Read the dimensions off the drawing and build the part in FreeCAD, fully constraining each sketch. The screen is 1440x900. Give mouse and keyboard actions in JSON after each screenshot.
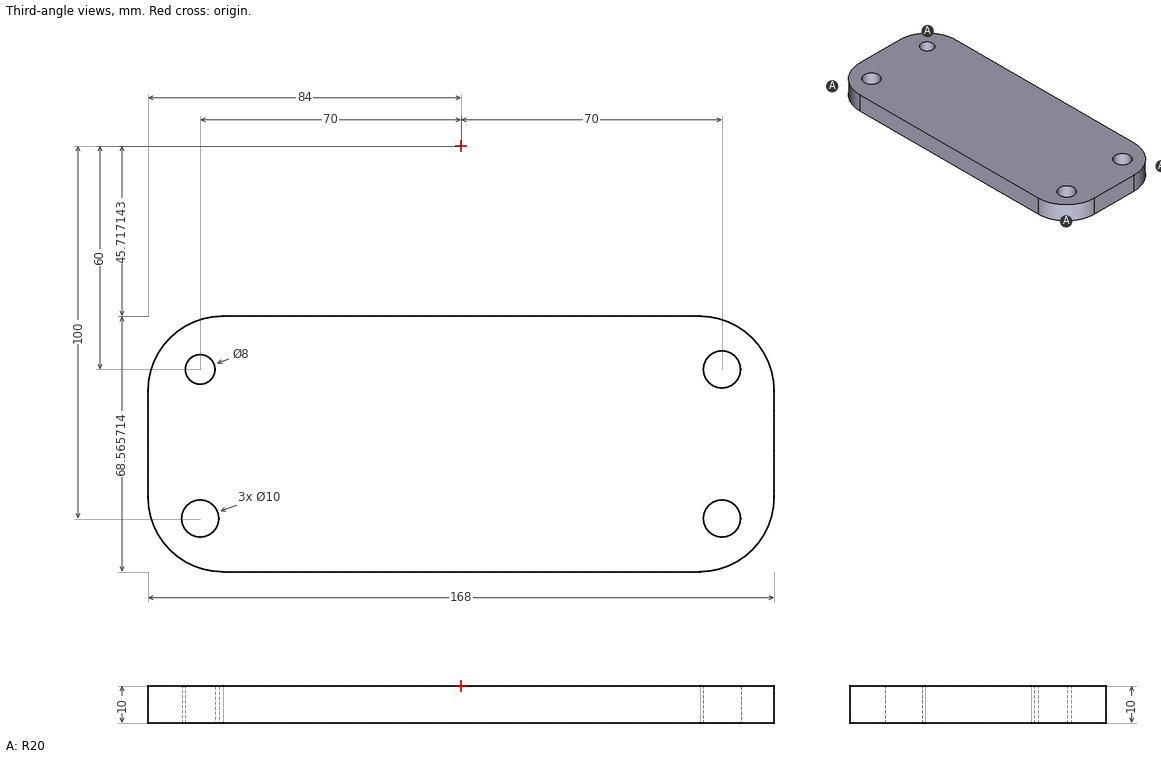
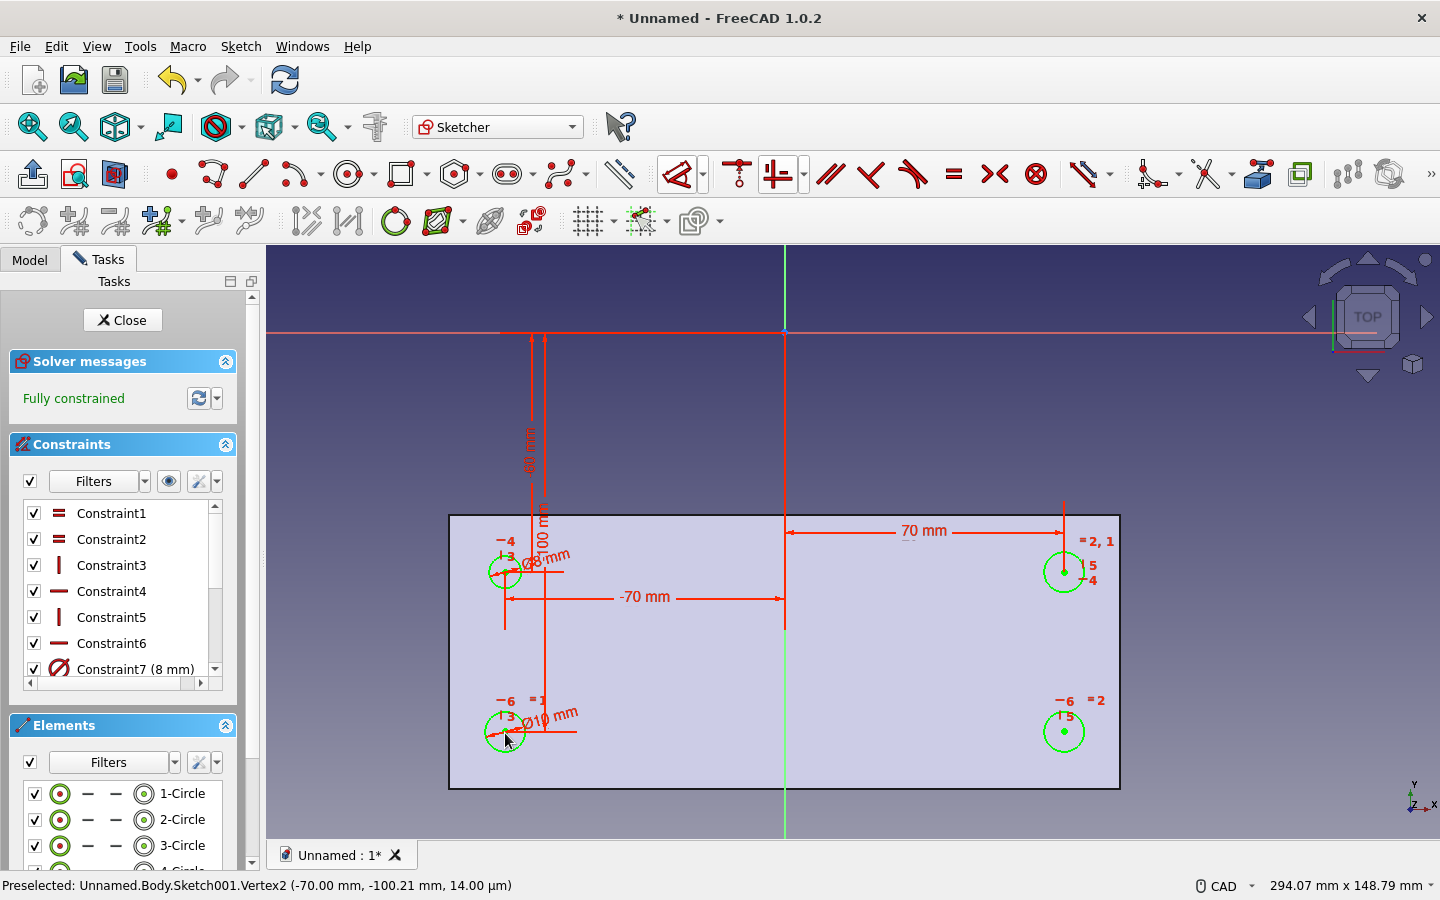
{"action": "left_click", "coordinate": [123, 320]}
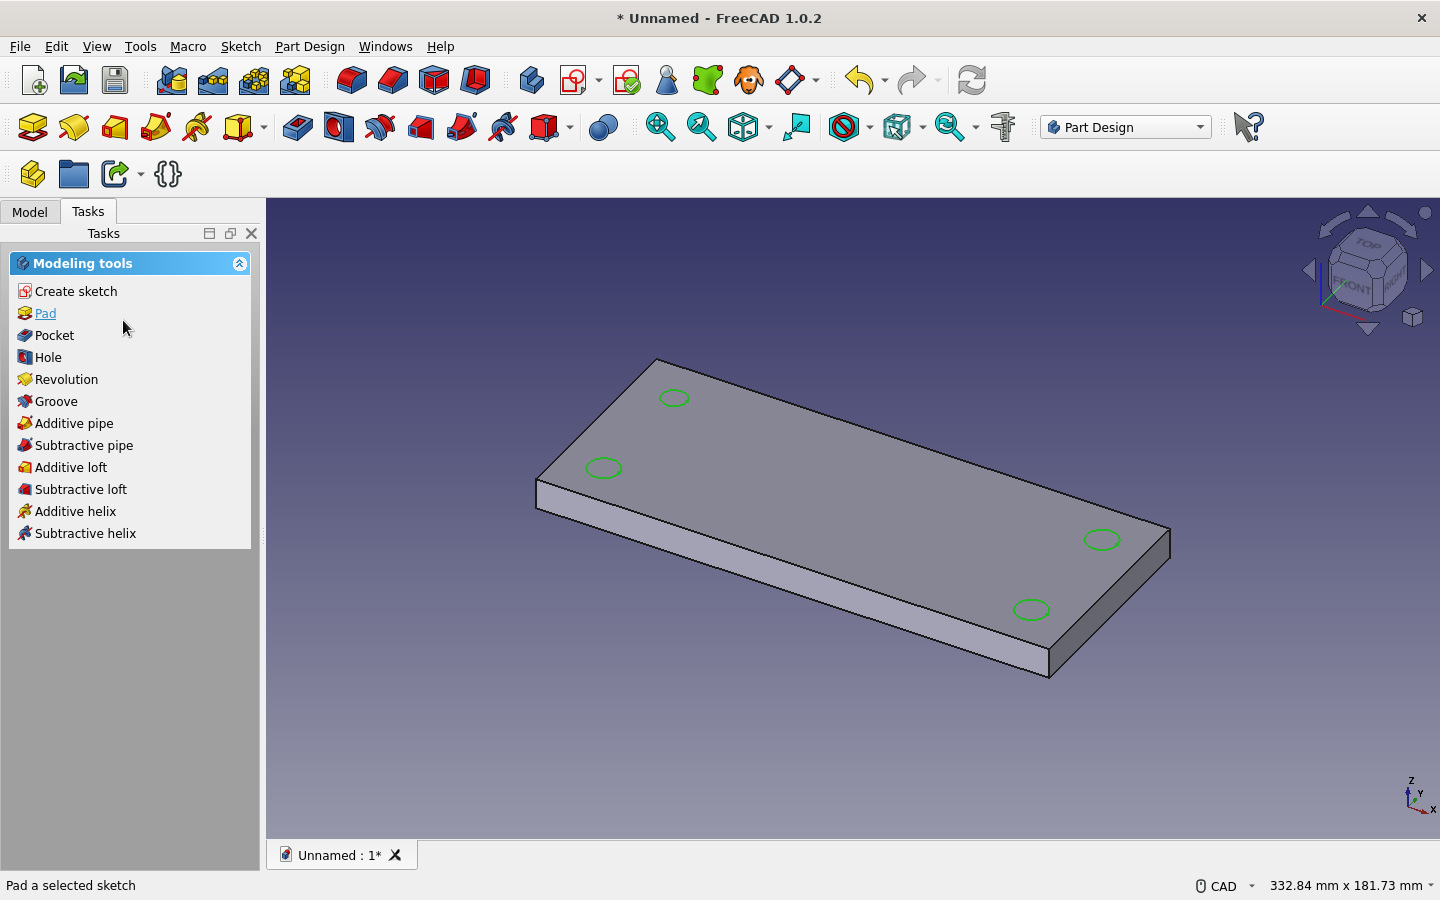
{"action": "left_click", "coordinate": [298, 128]}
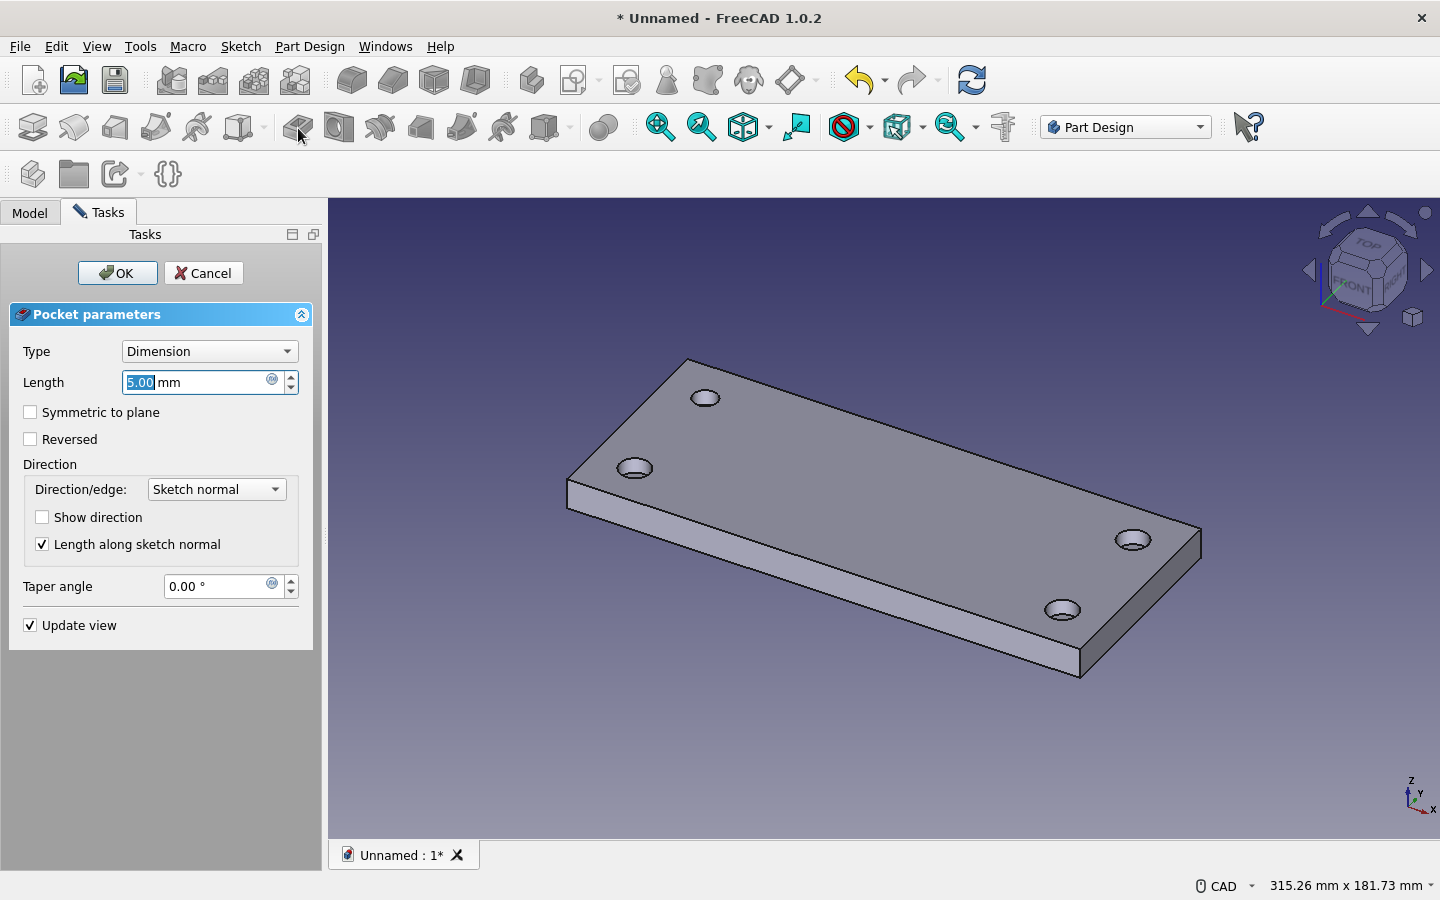
{"action": "type", "text": "10"}
{"action": "key", "text": "Tab"}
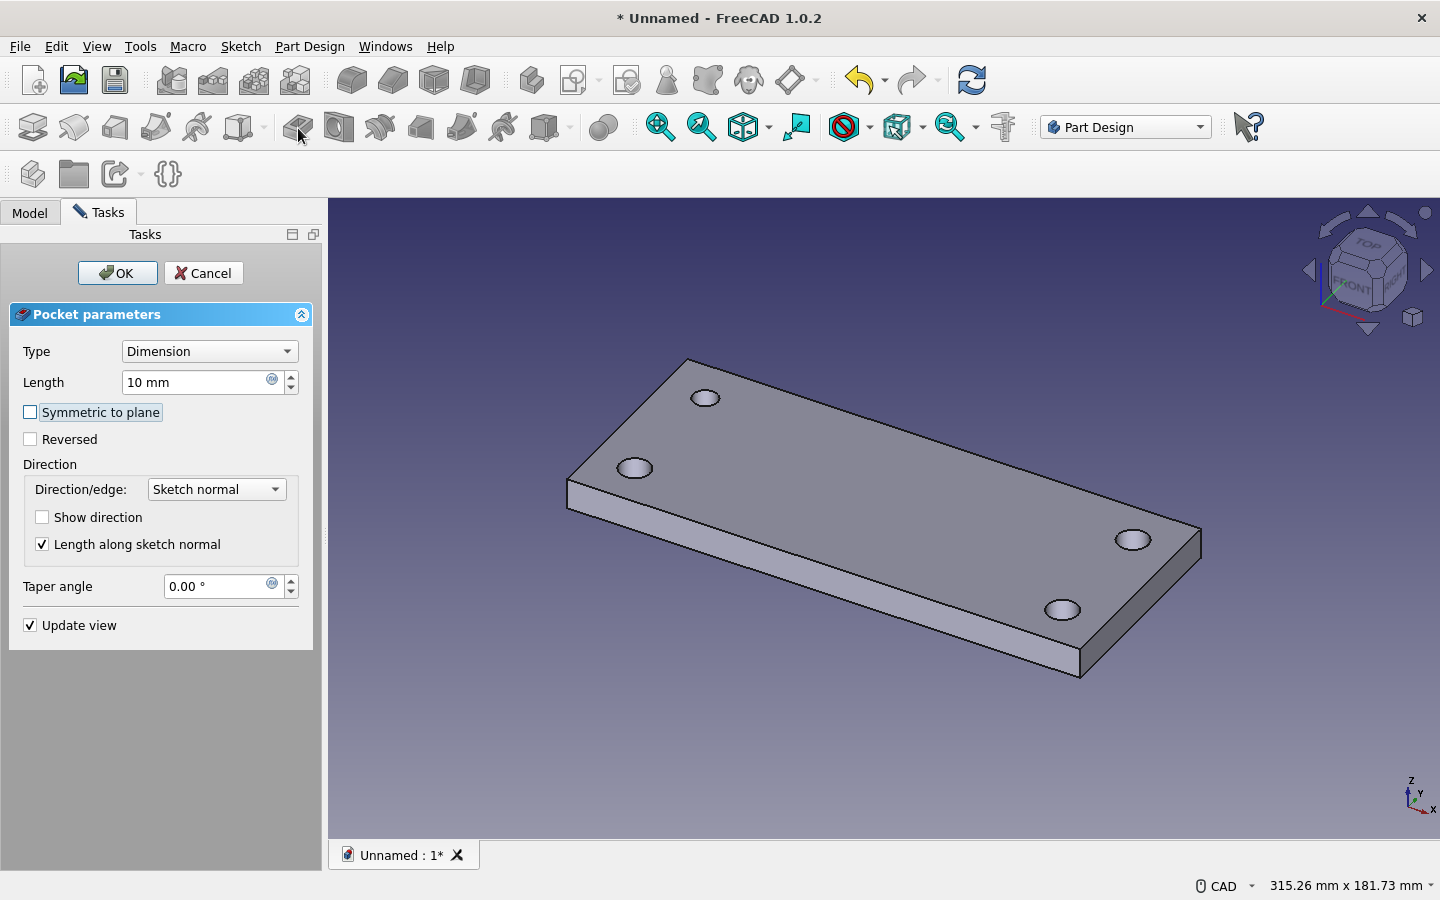
{"action": "left_click", "coordinate": [118, 273]}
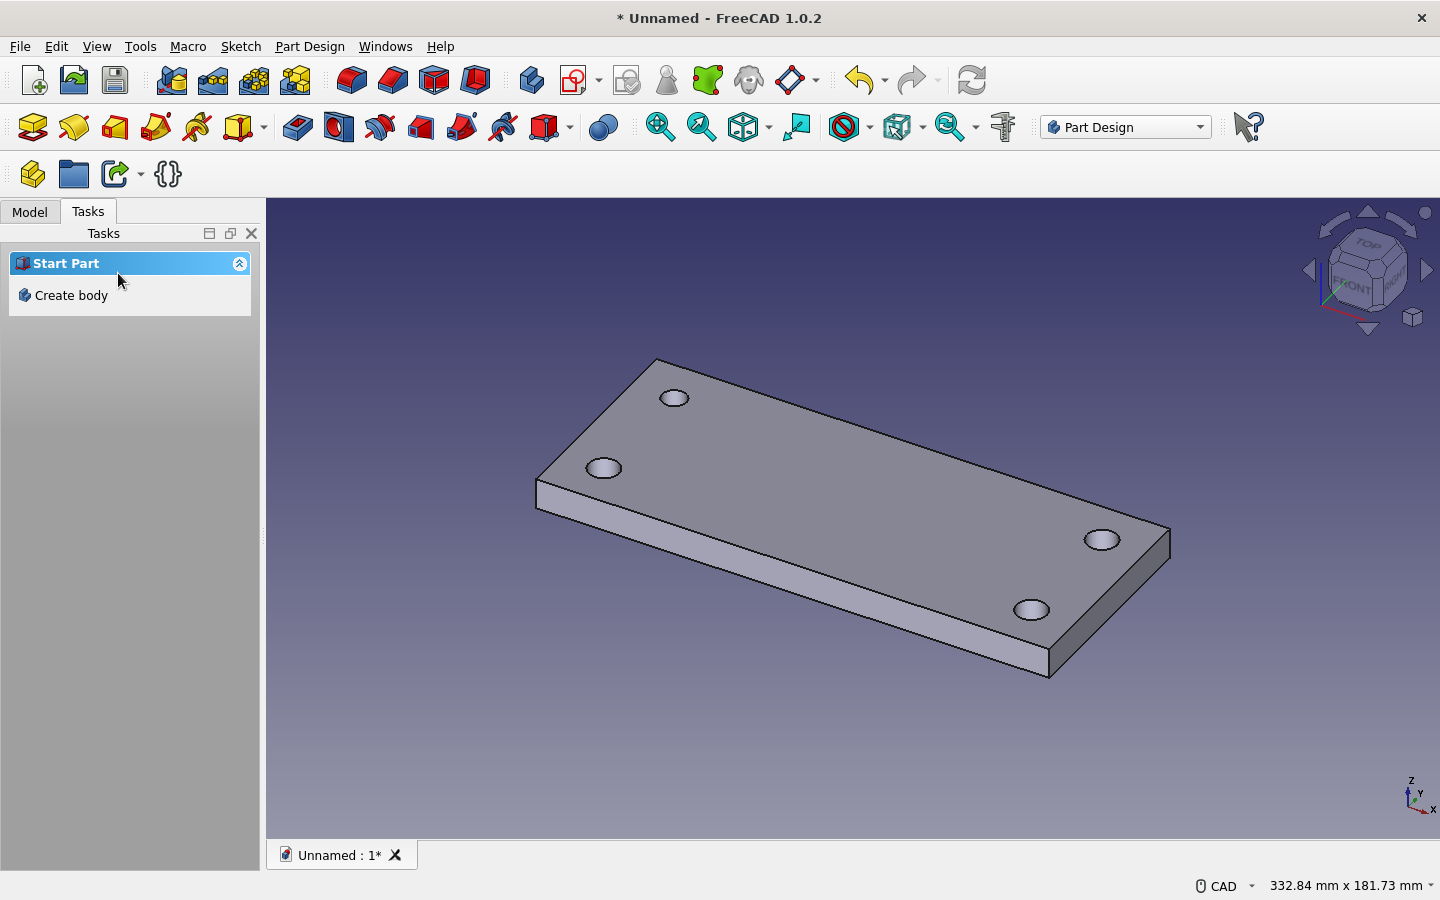
{"action": "left_click", "coordinate": [1049, 663]}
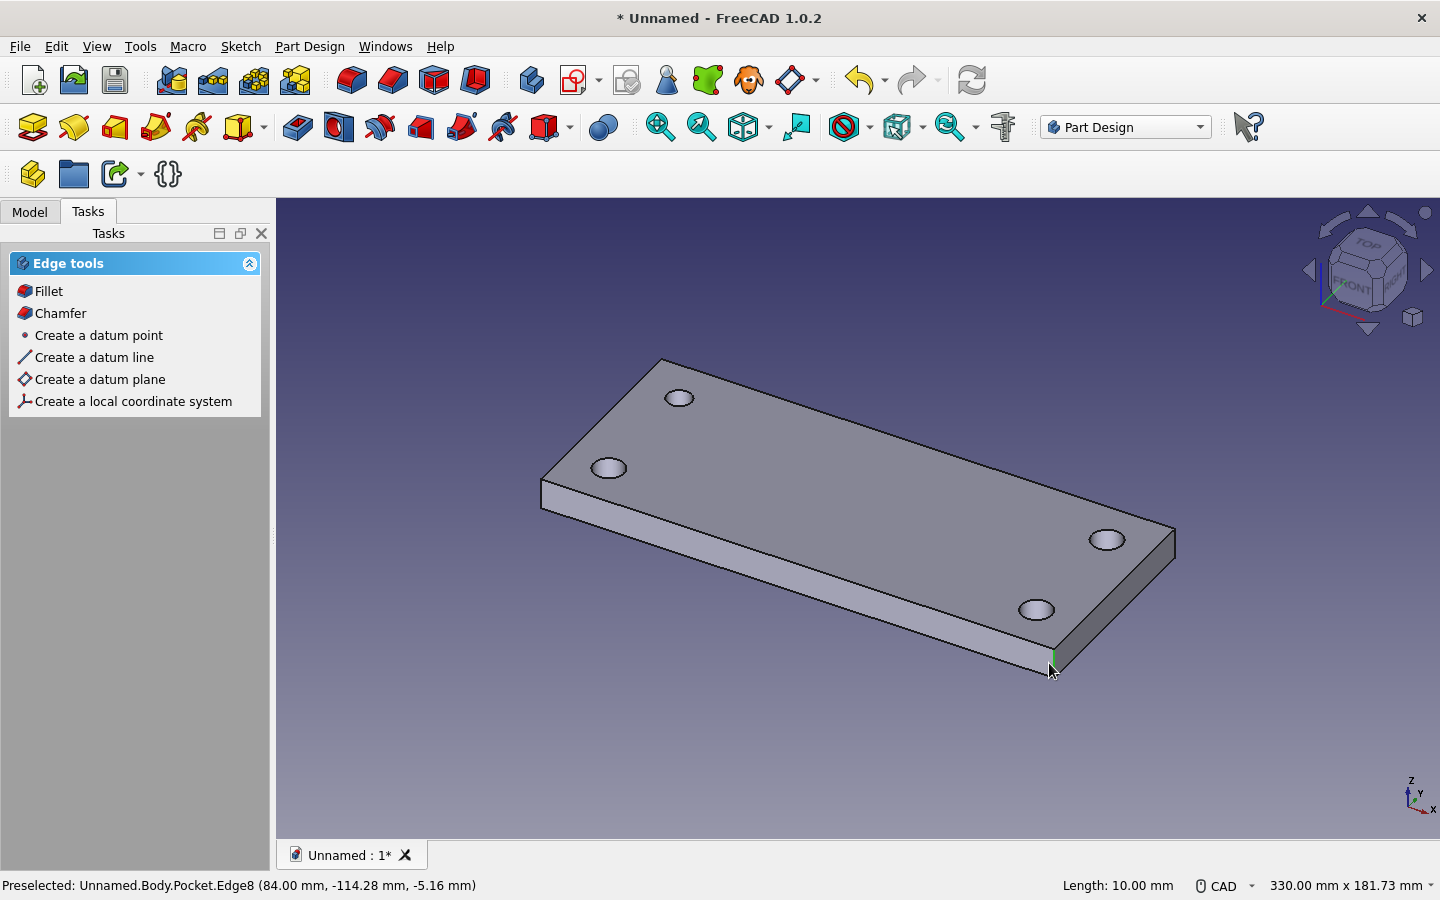
{"action": "key", "text": "0"}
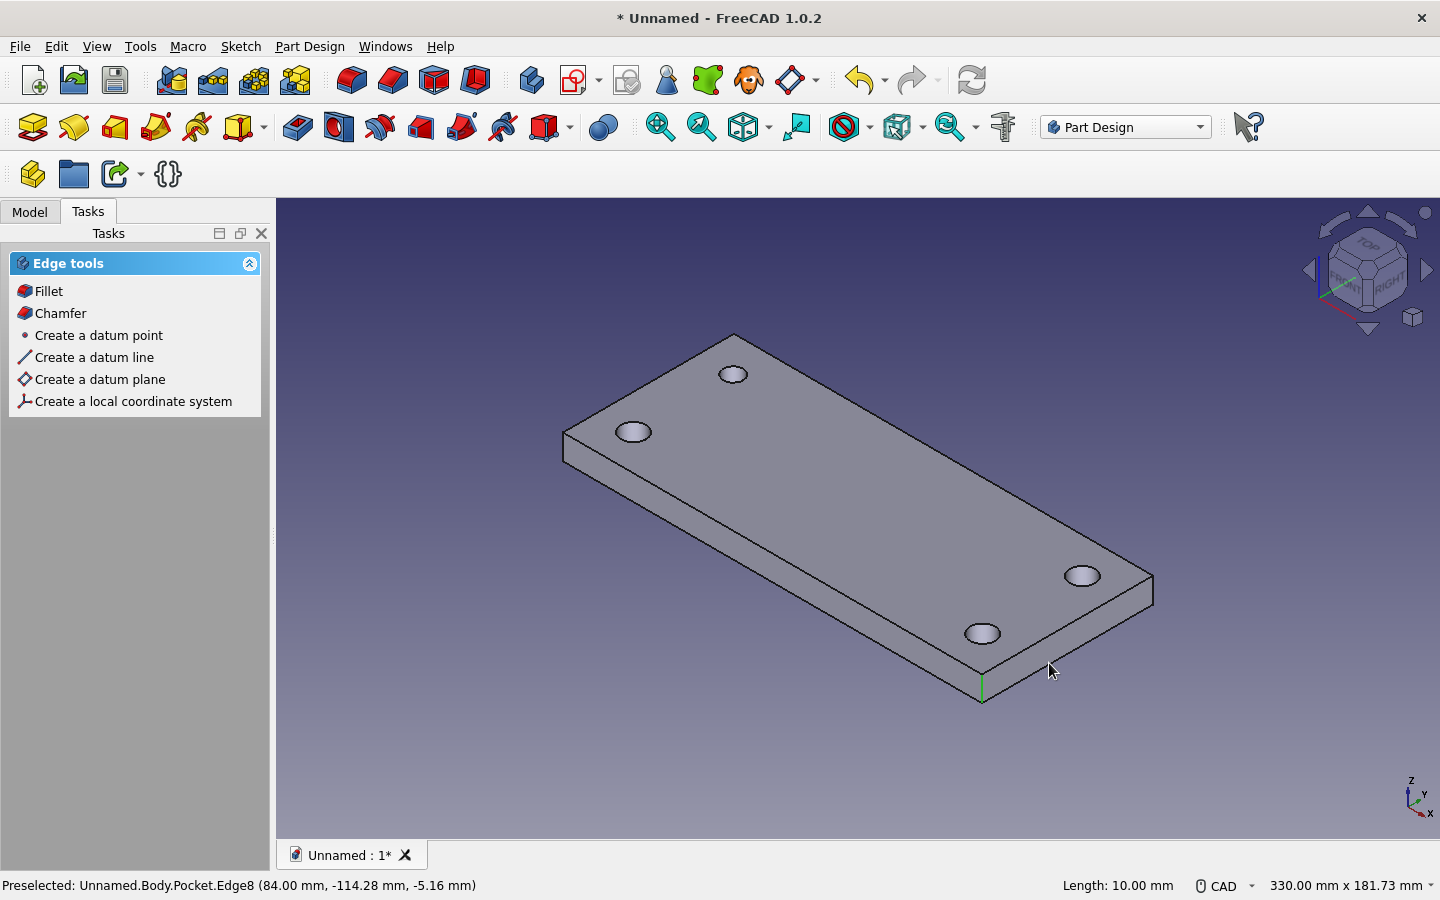
{"action": "key", "text": "2"}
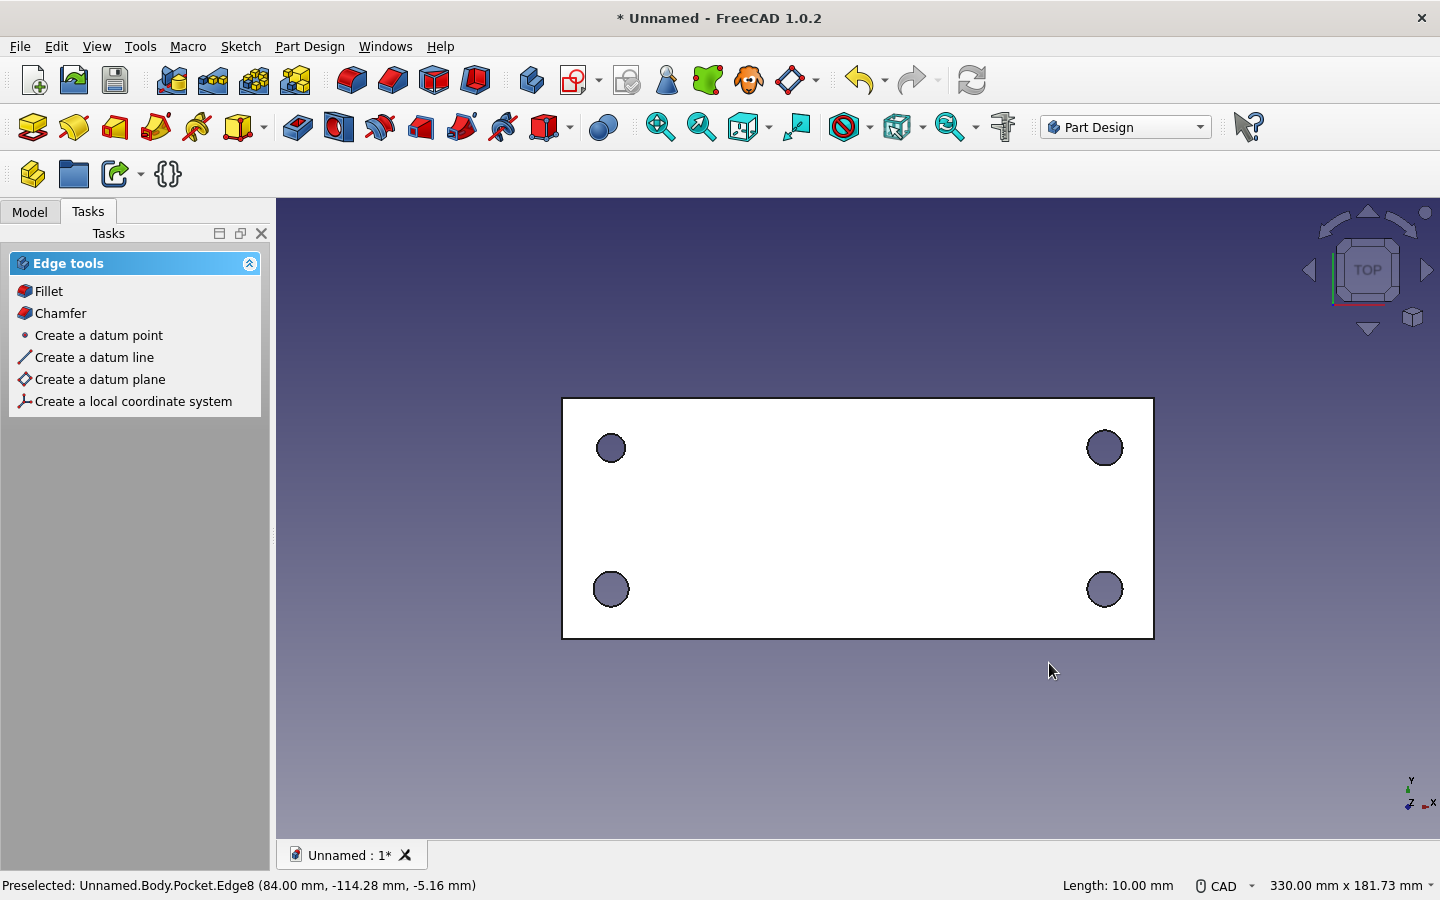
{"action": "key", "text": "1"}